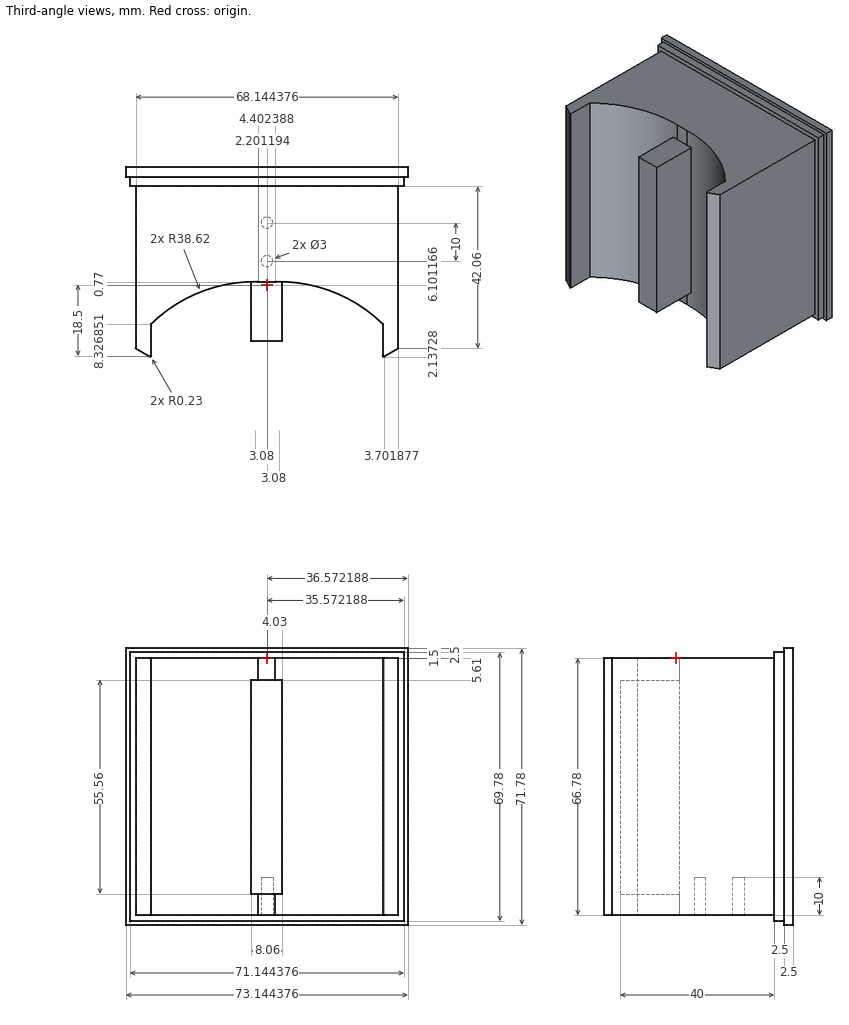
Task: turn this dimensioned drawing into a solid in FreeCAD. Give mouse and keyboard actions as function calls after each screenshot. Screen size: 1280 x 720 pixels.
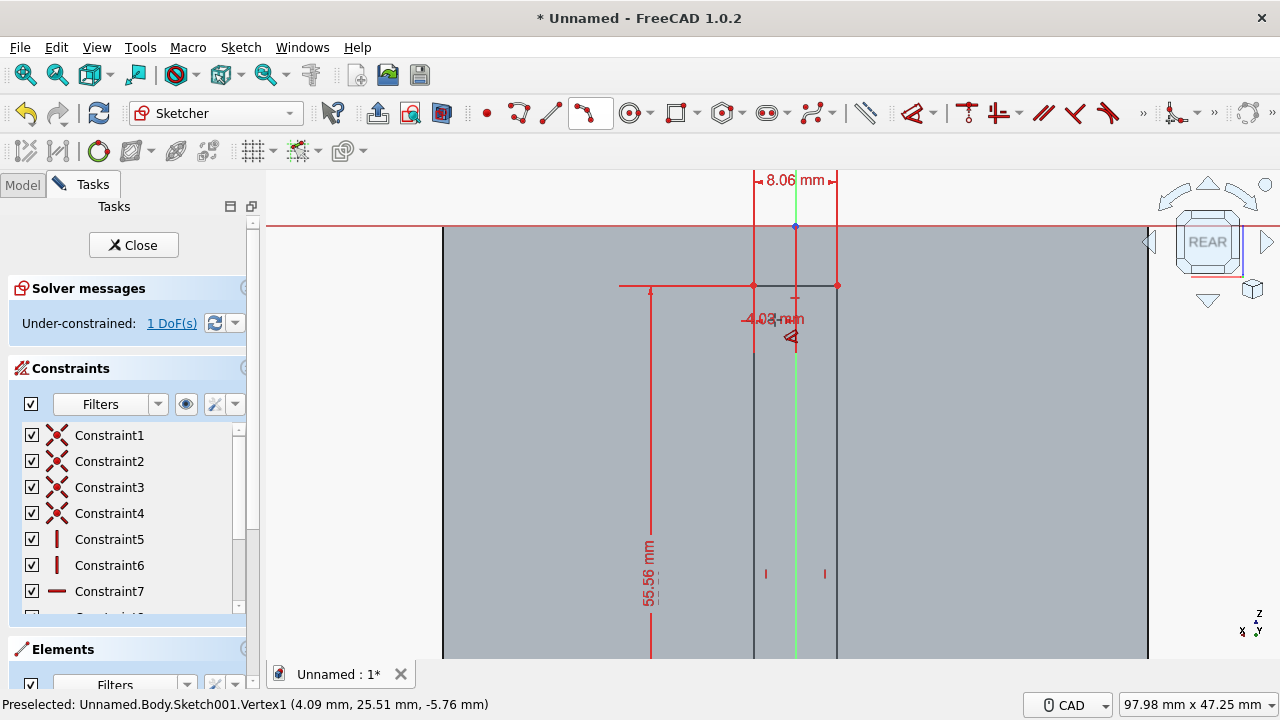
click(754, 286)
click(720, 256)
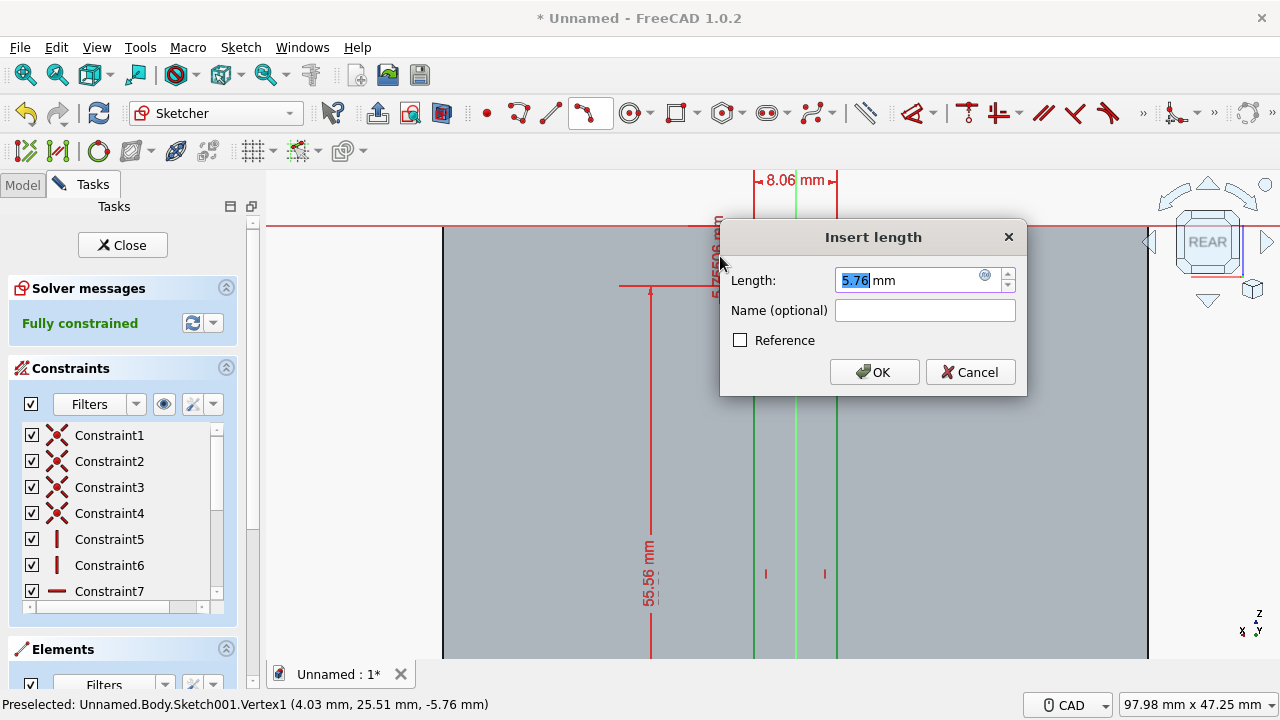
text(5.61)
key(Return)
key(Escape)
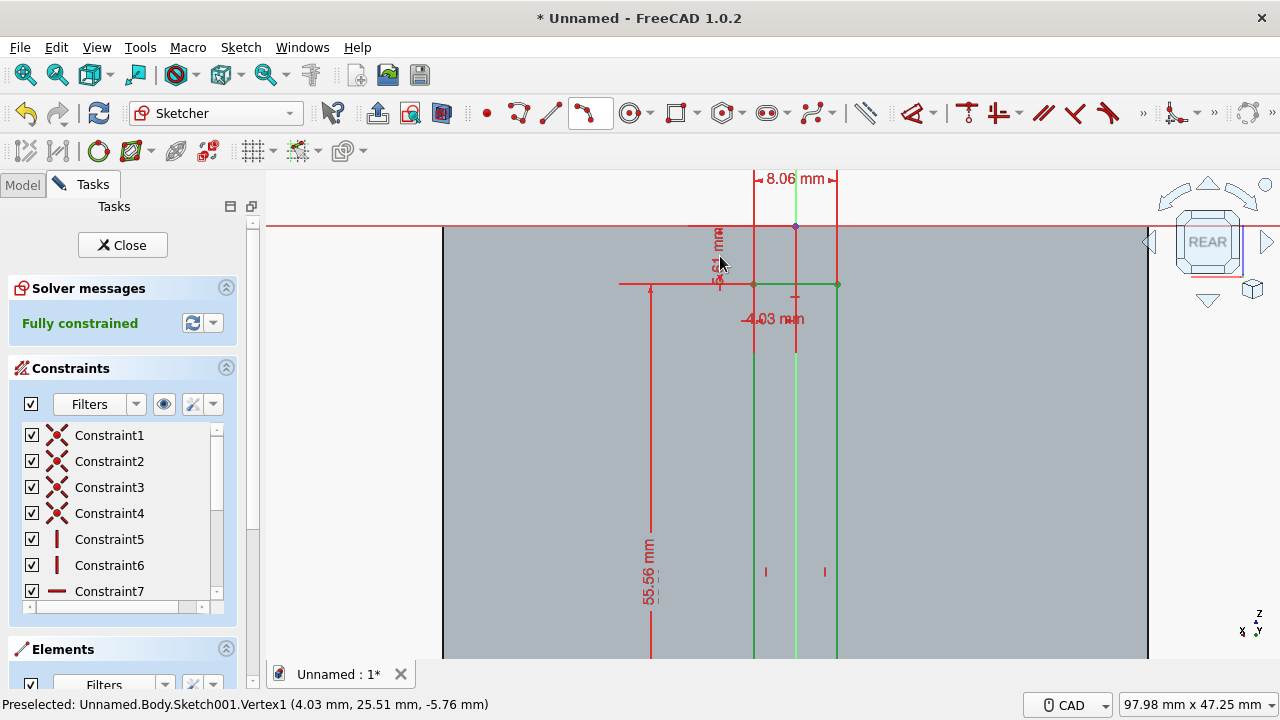
click(123, 245)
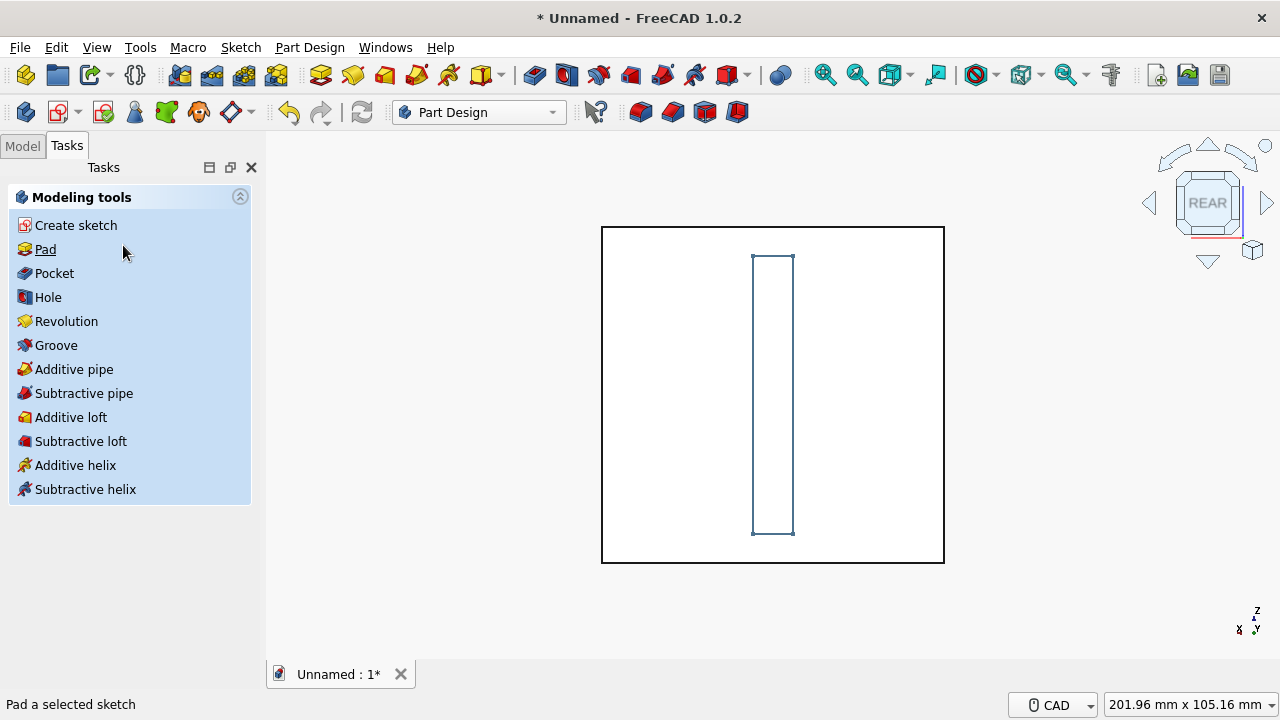
click(322, 76)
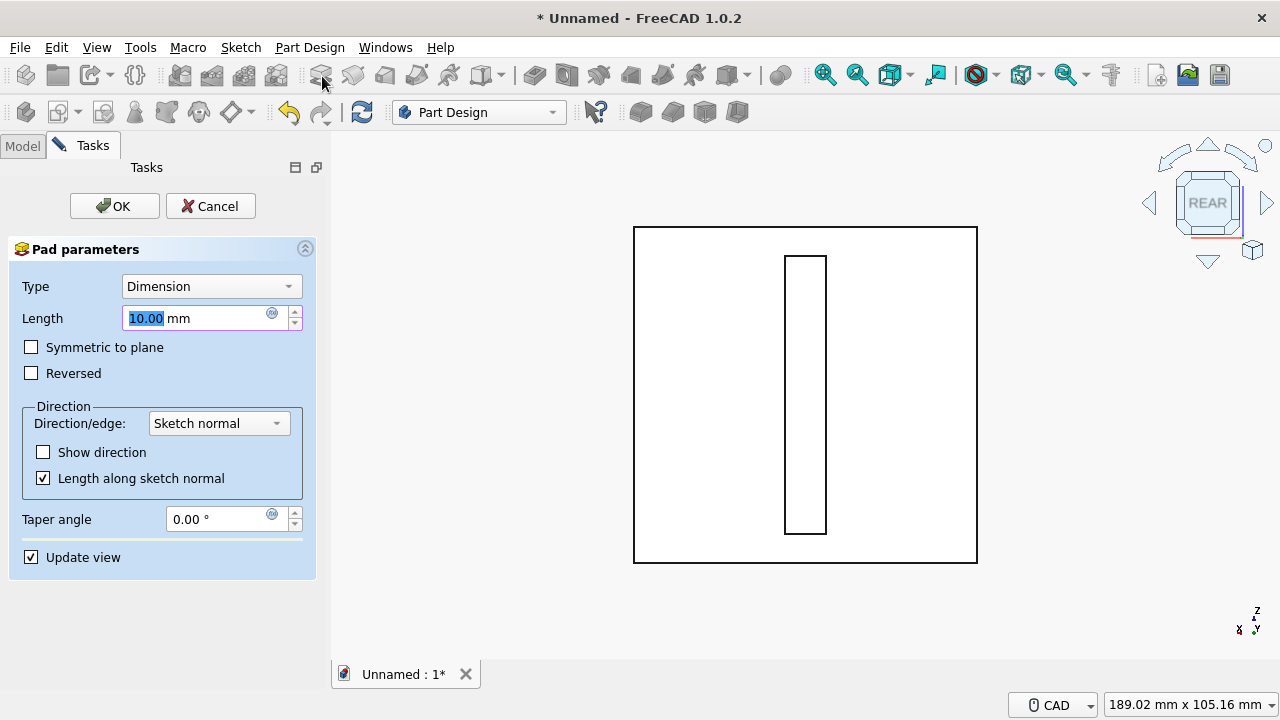
text(40)
key(Tab)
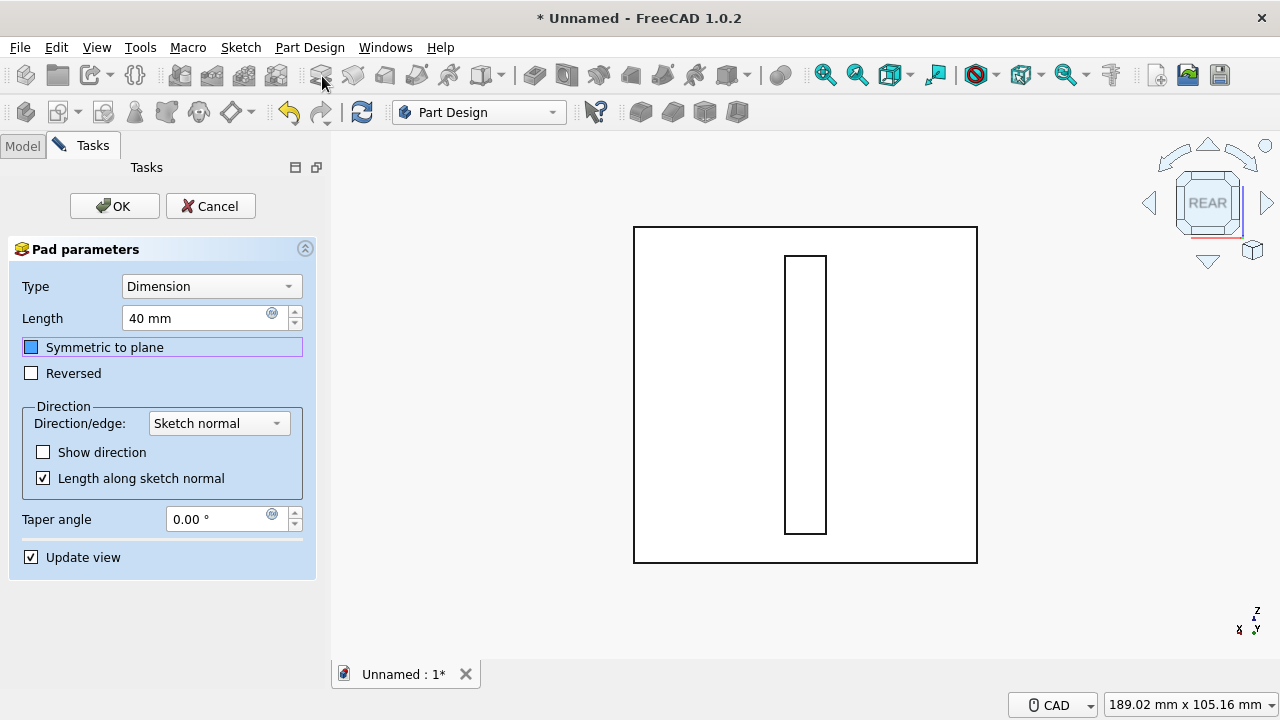
click(30, 373)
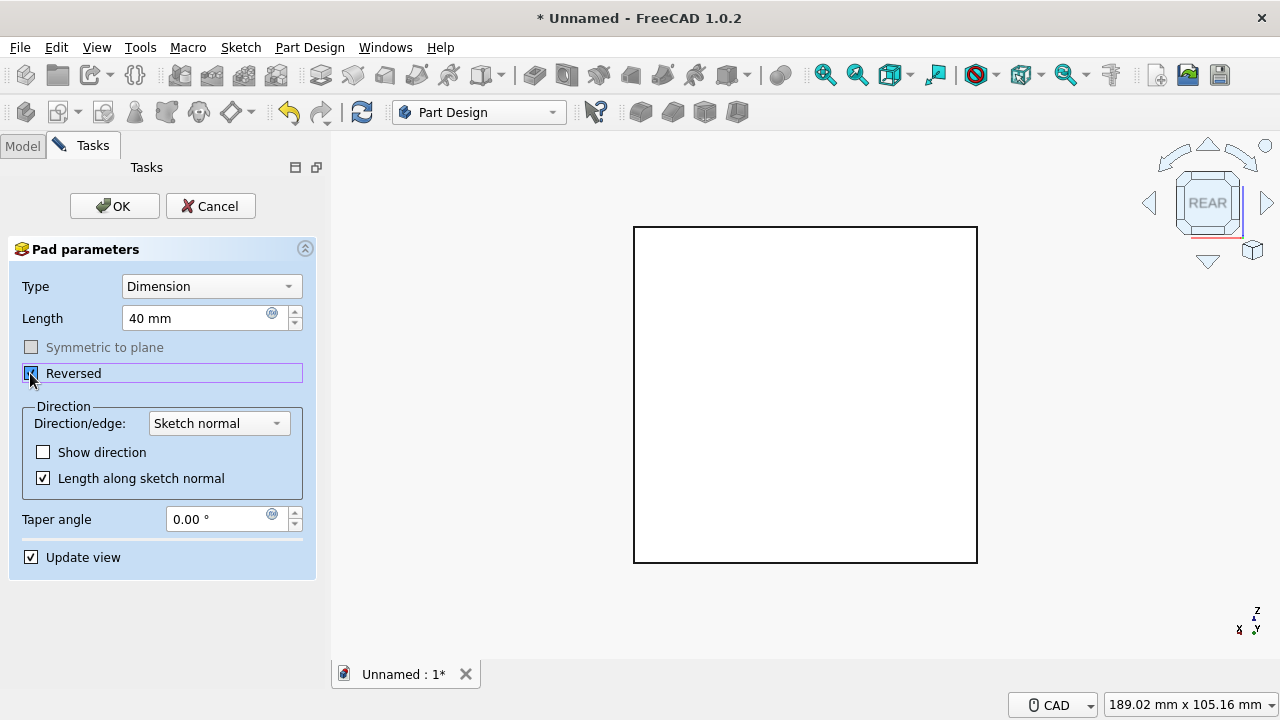
click(115, 206)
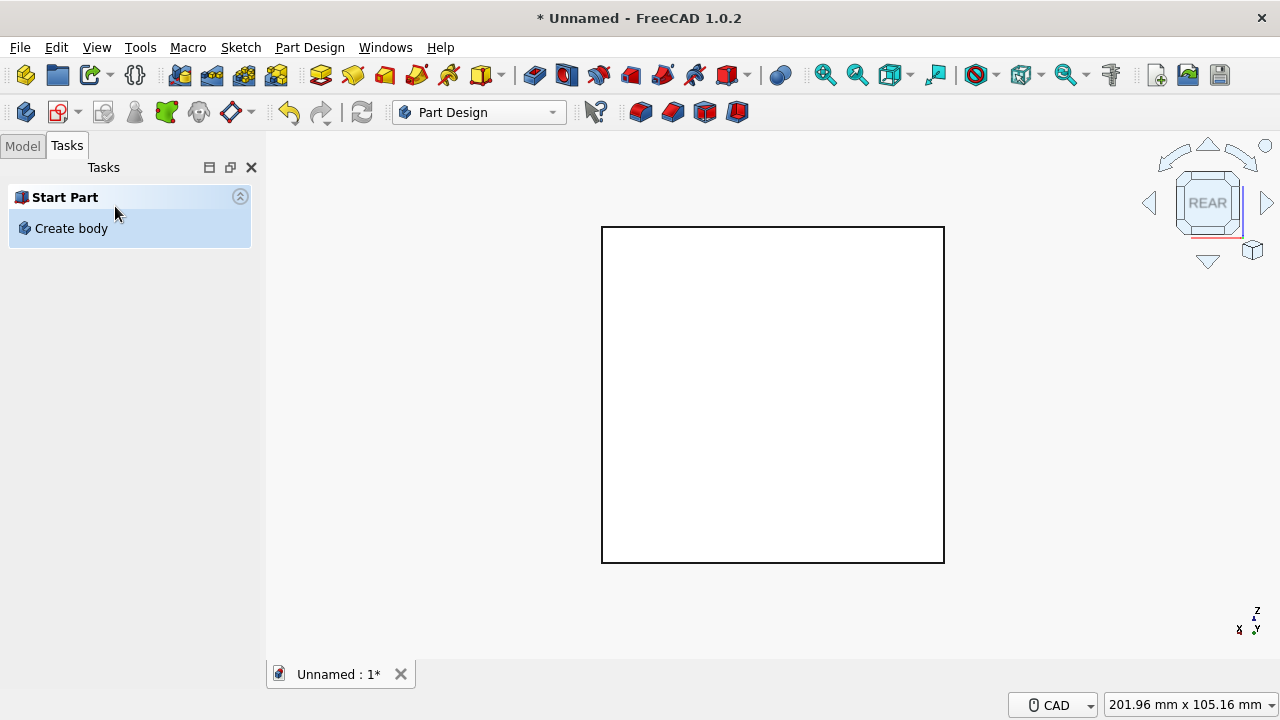
click(773, 394)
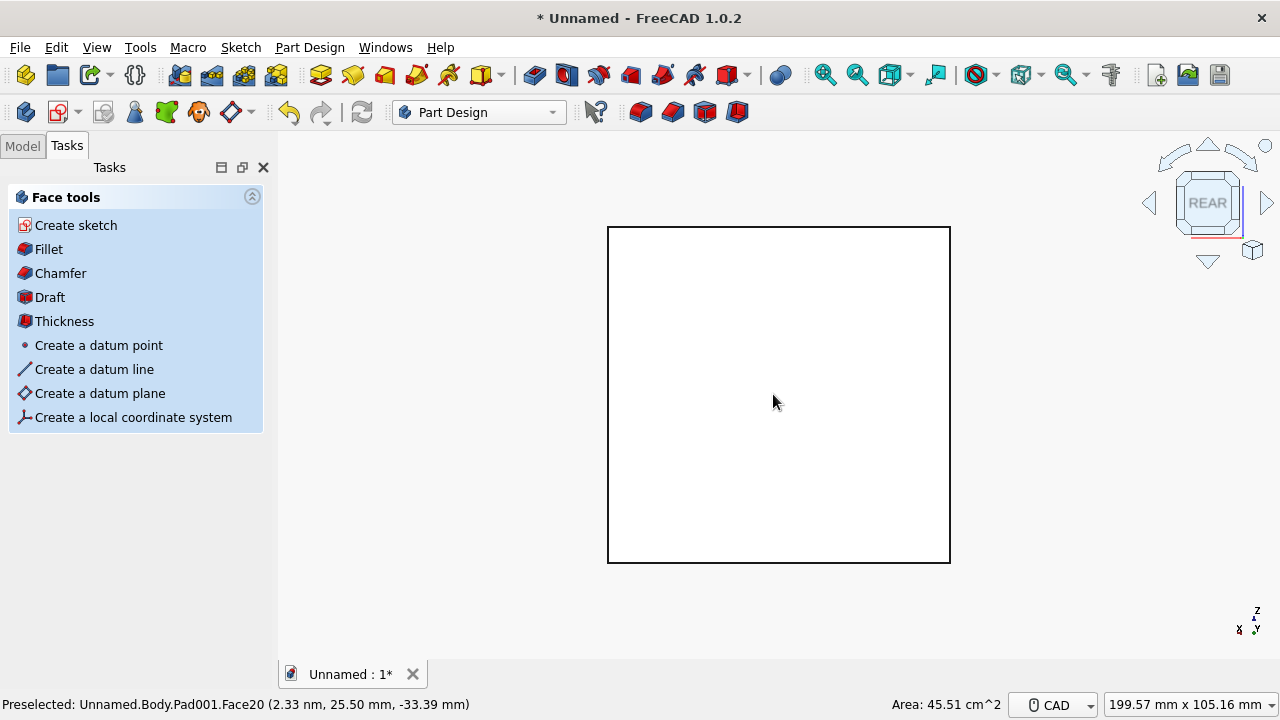
click(58, 112)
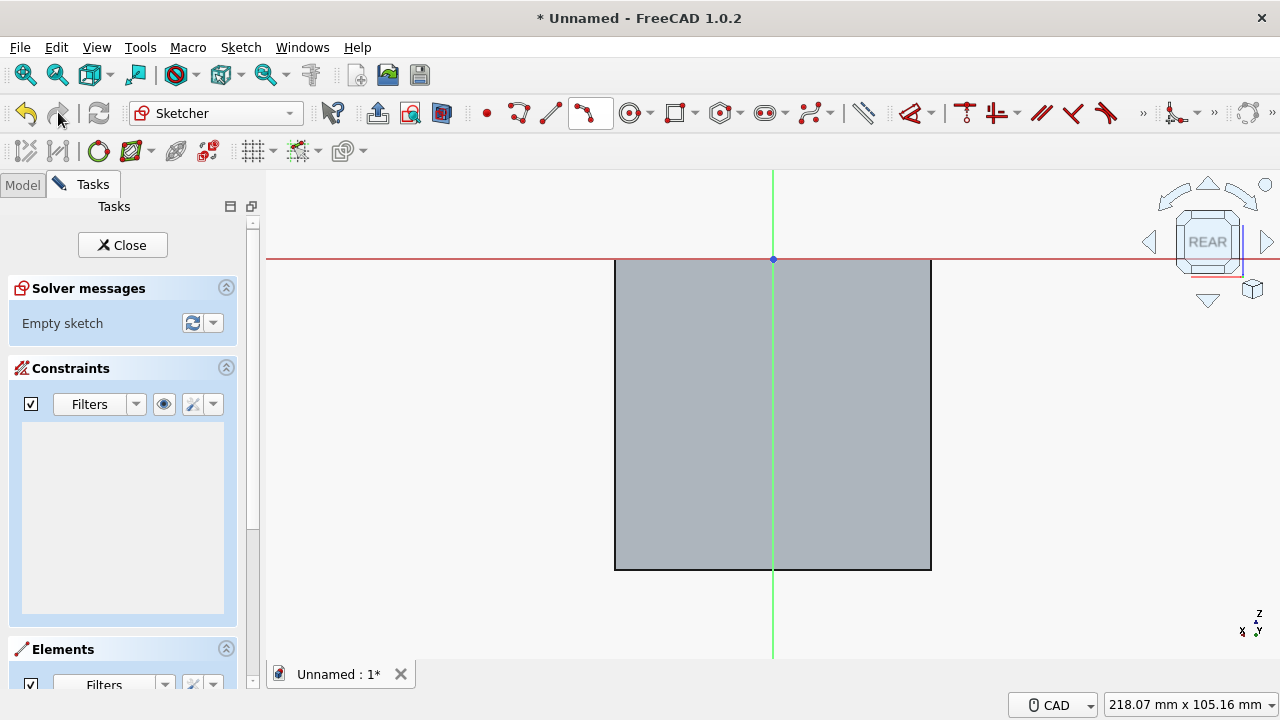
click(676, 114)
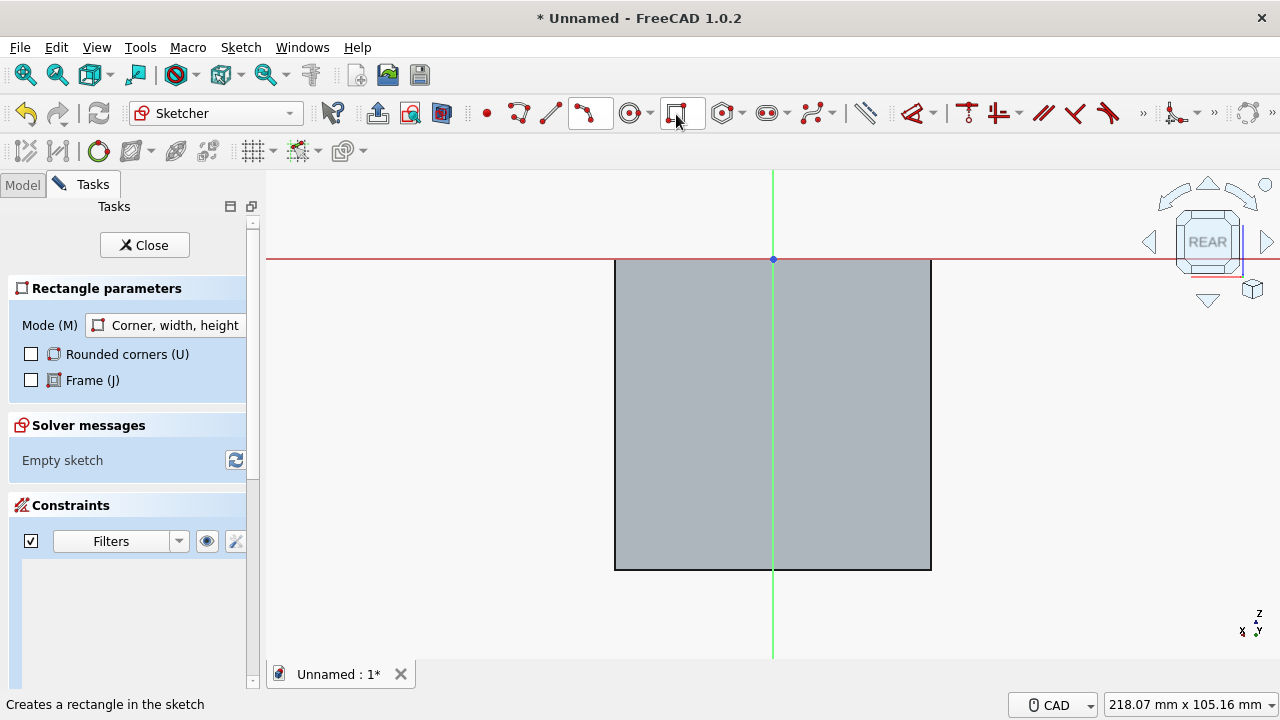
scroll(608, 252, up, 5)